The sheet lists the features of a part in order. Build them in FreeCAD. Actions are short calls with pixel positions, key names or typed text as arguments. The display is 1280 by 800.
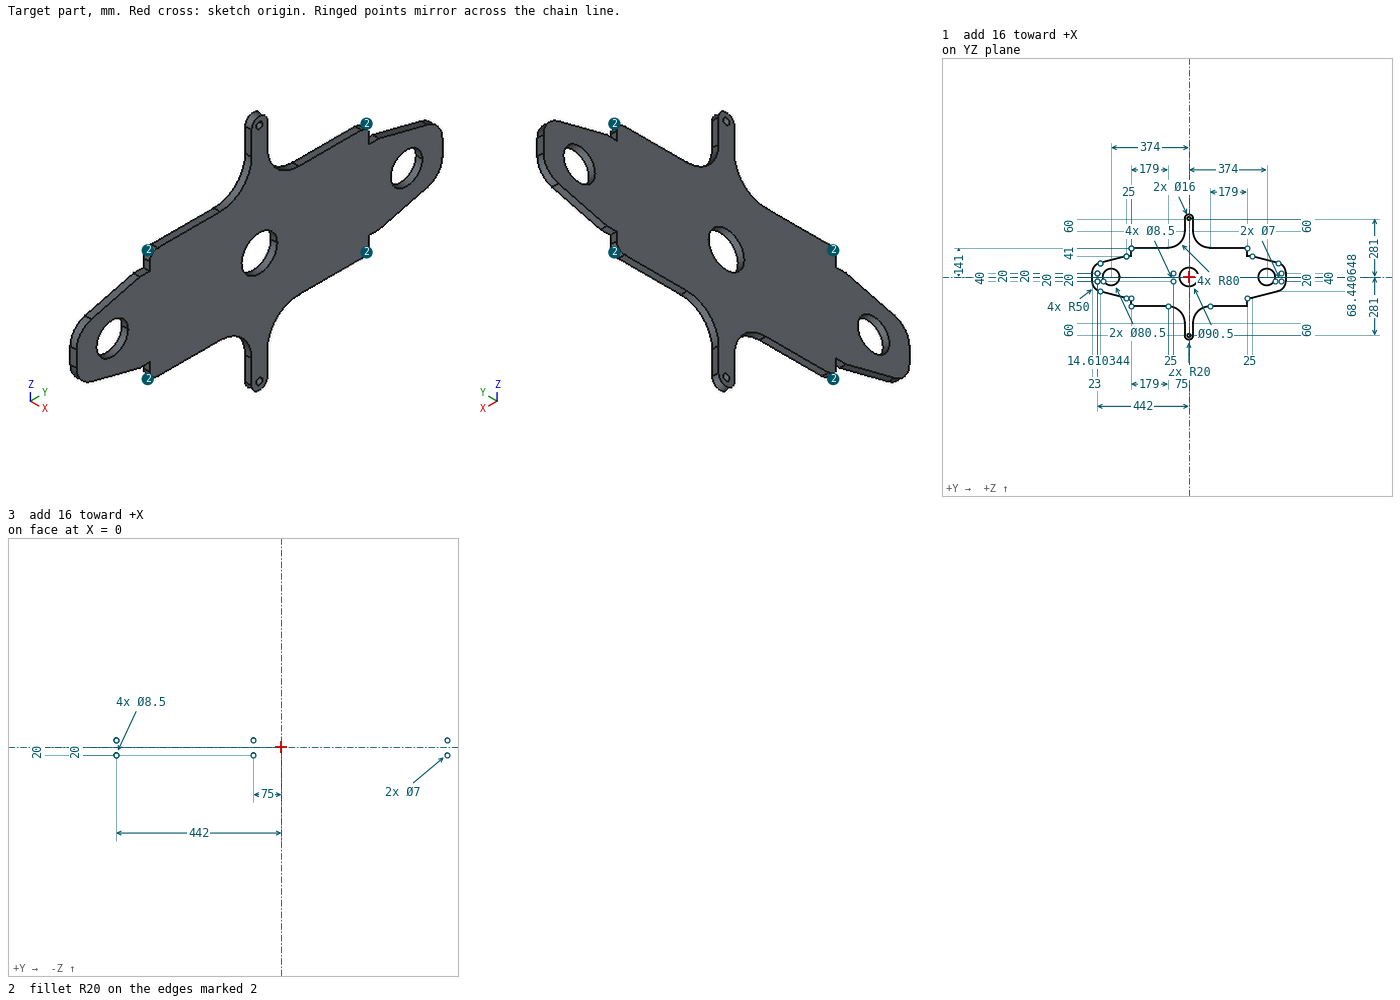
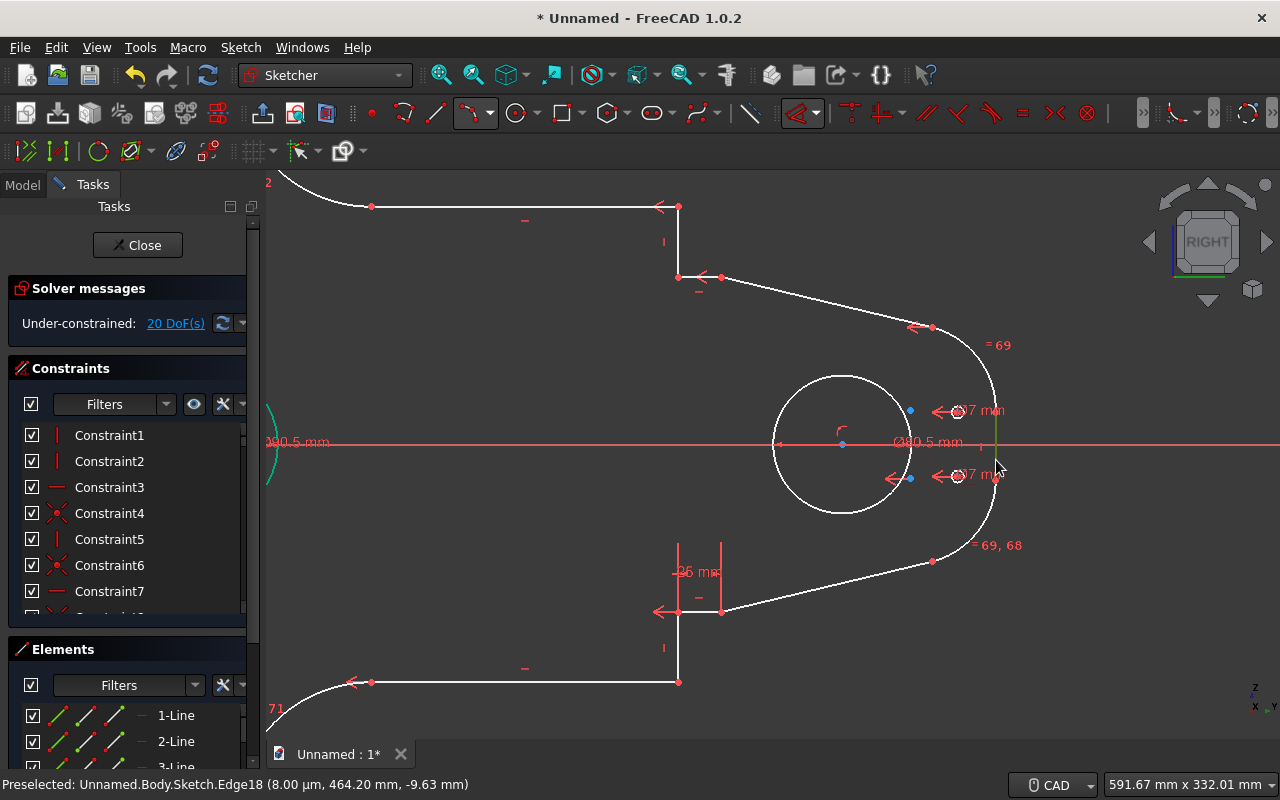
key(i)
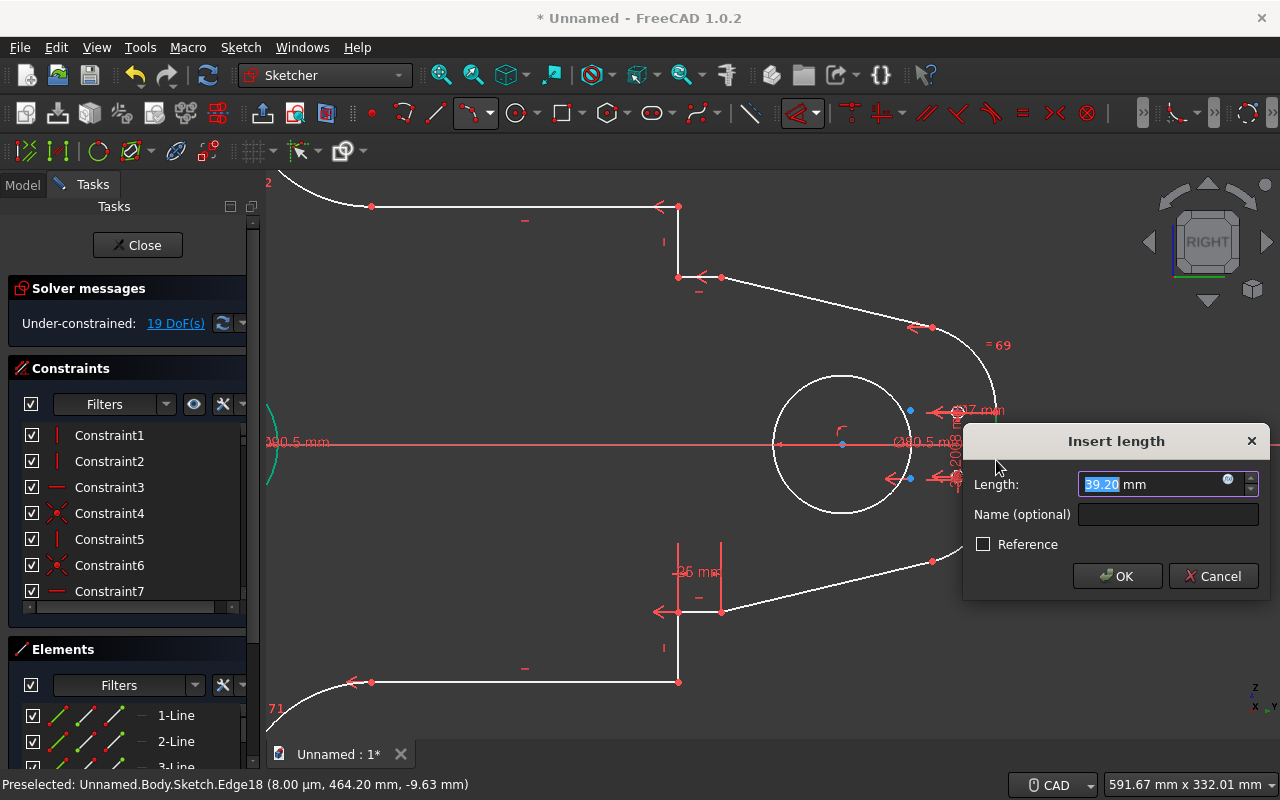
text(40)
key(Return)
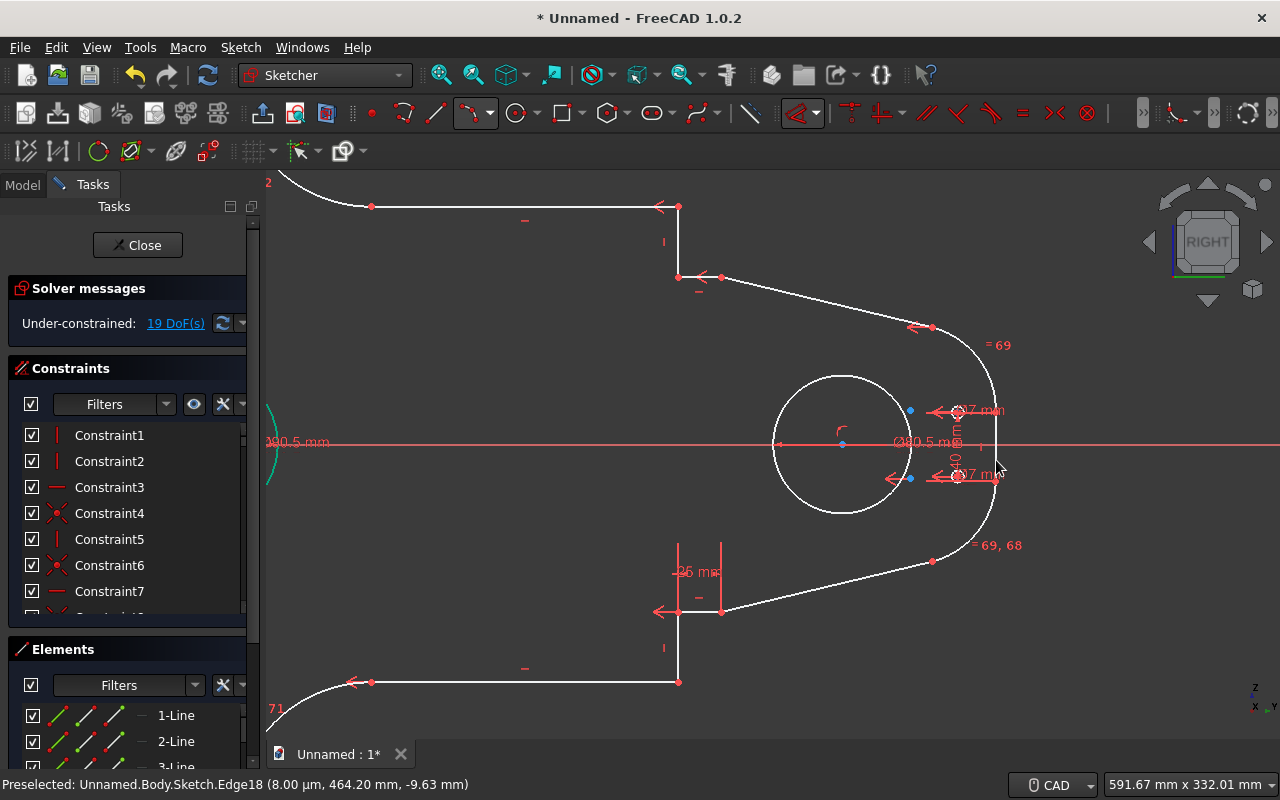
scroll(998, 460, down, 5)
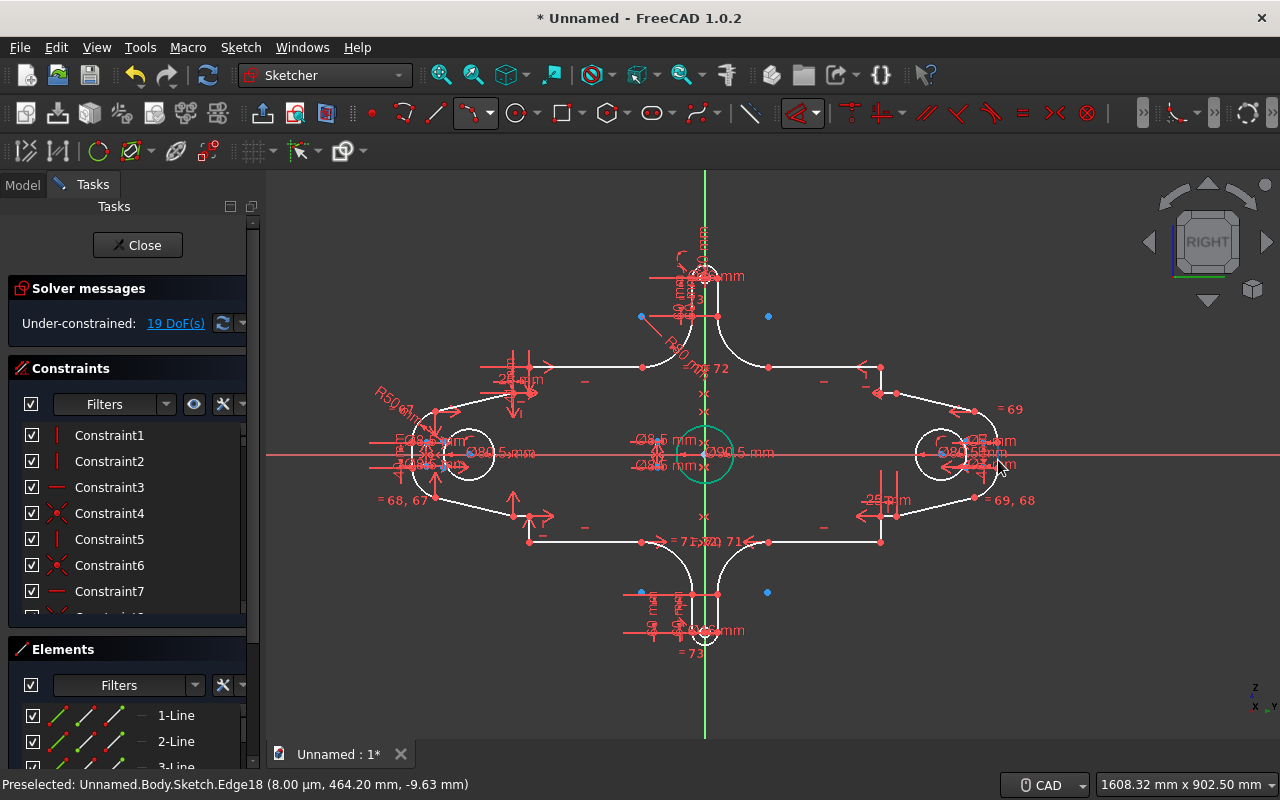
scroll(426, 466, up, 6)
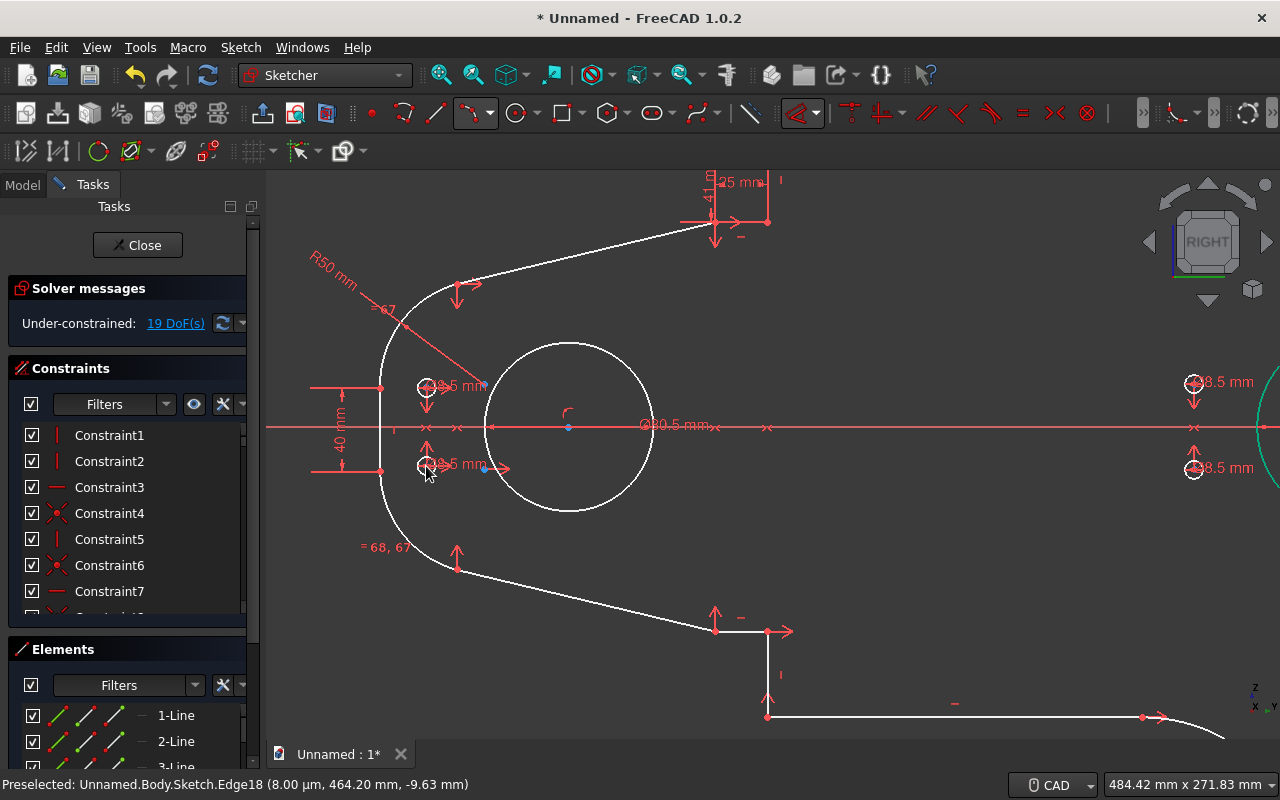
click(427, 466)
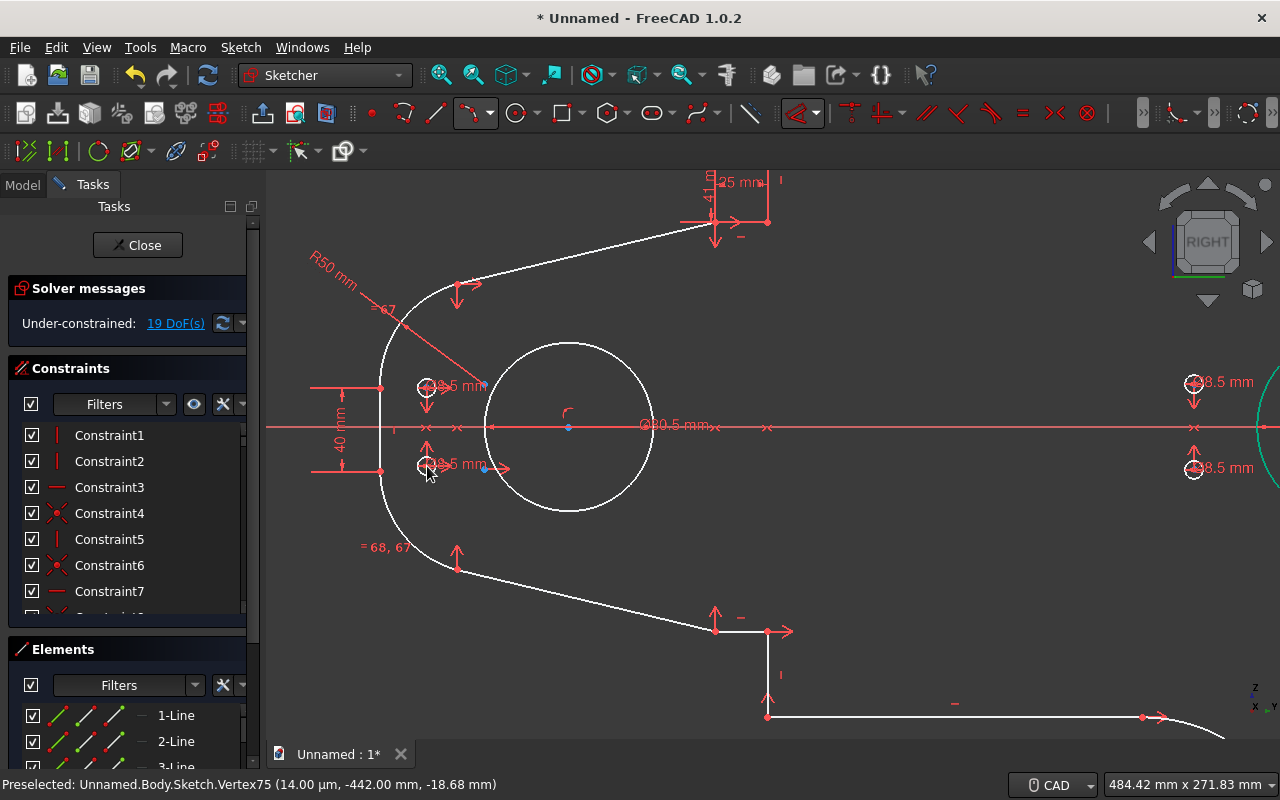
click(818, 114)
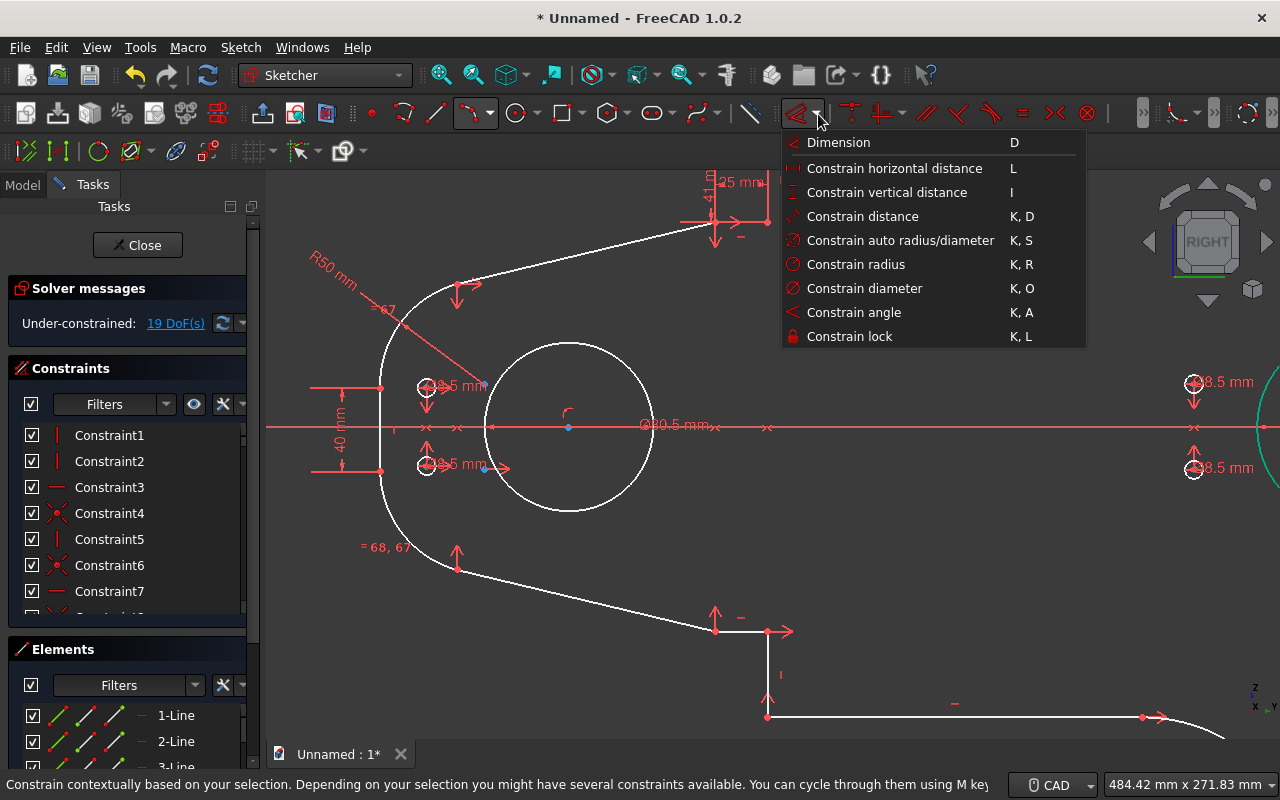
click(934, 192)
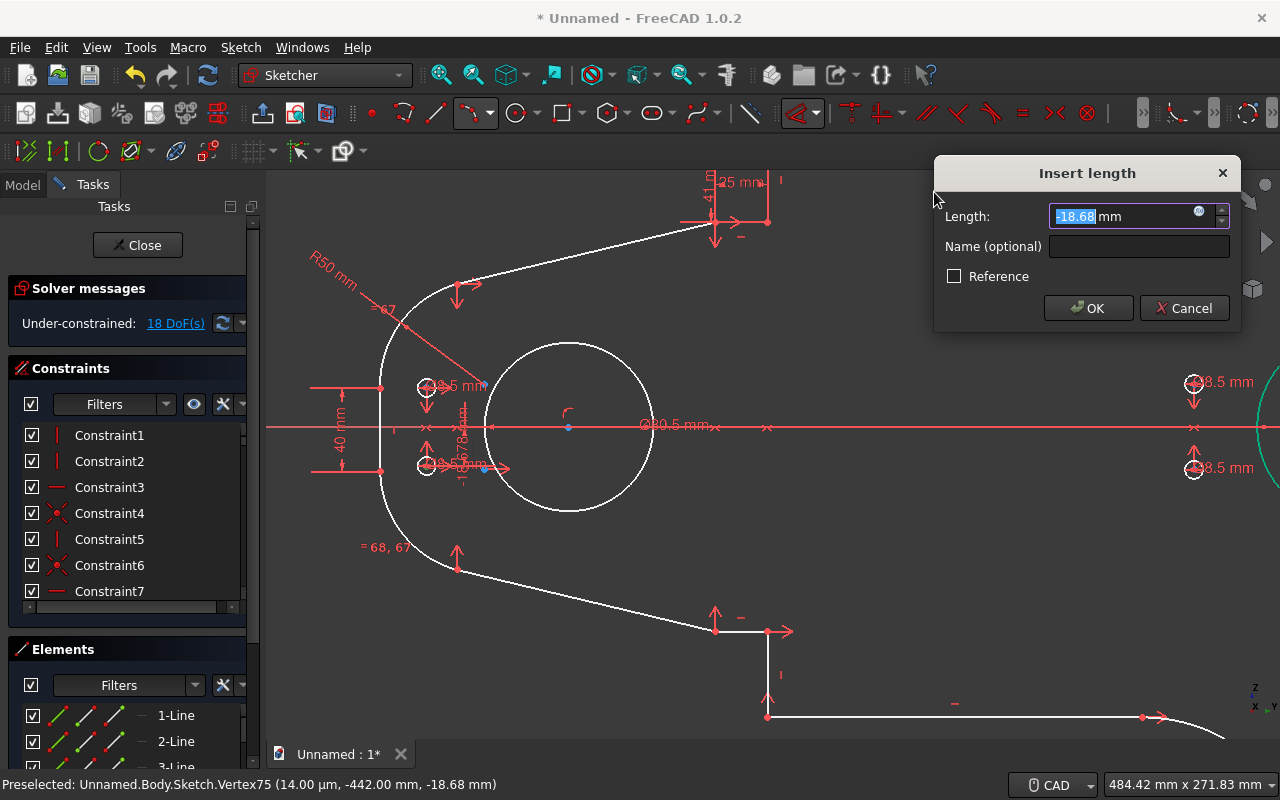
text(-20)
key(Return)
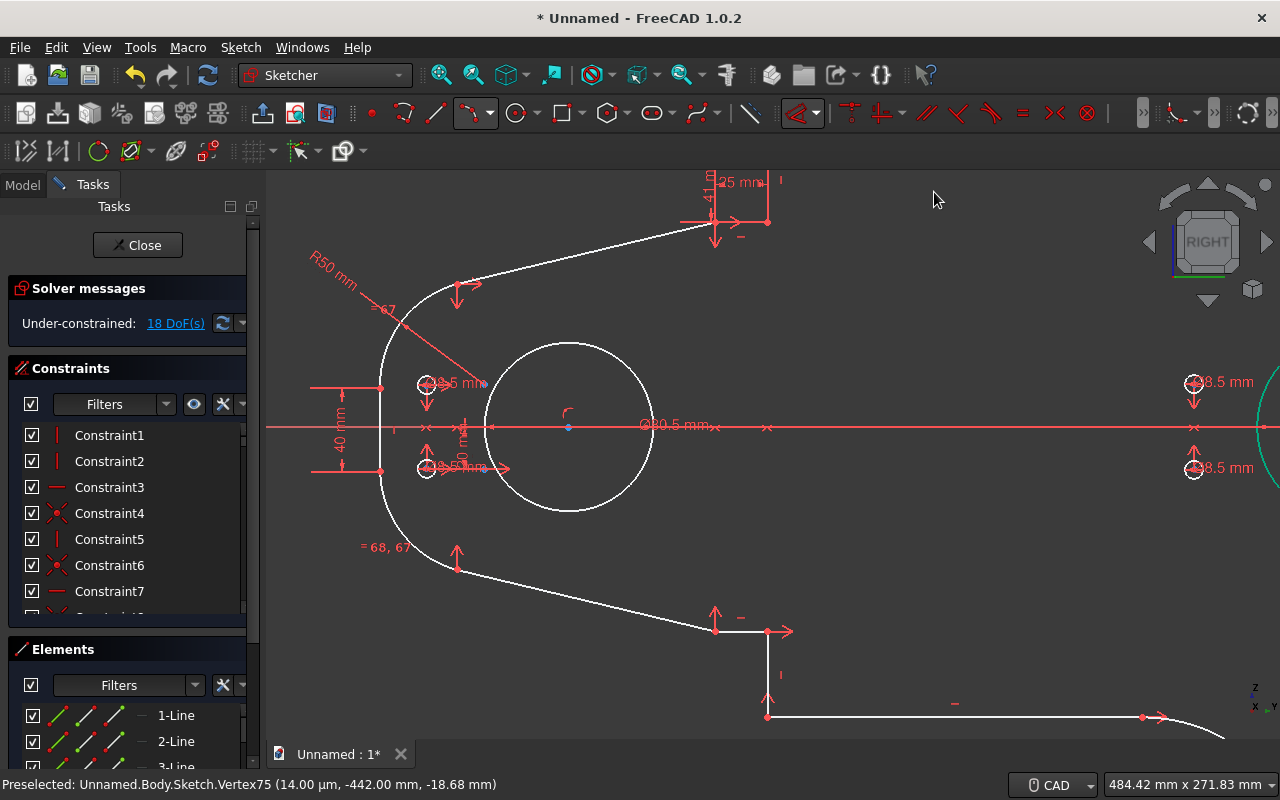
scroll(425, 466, down, 6)